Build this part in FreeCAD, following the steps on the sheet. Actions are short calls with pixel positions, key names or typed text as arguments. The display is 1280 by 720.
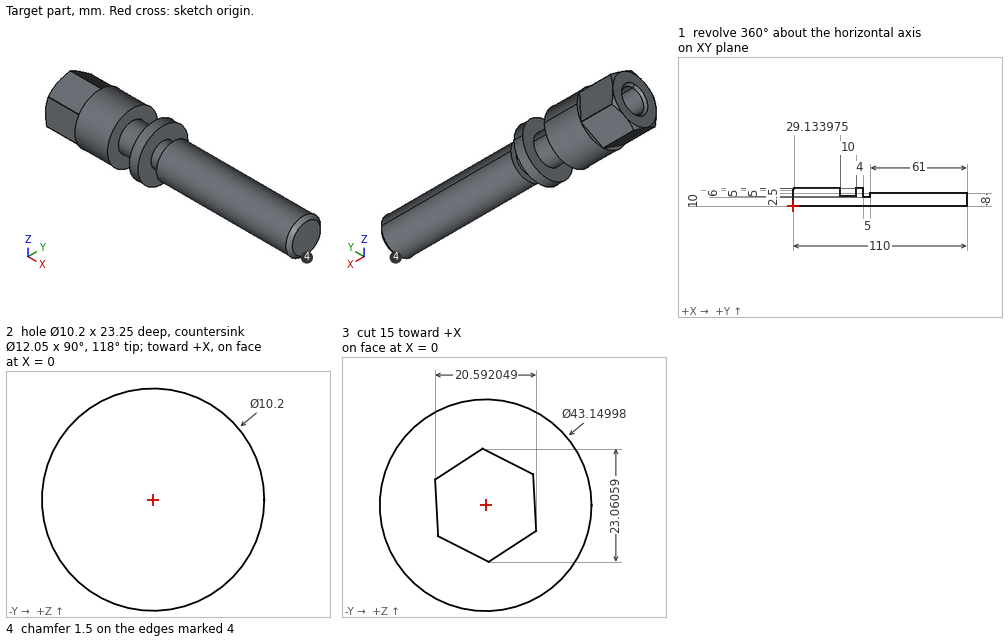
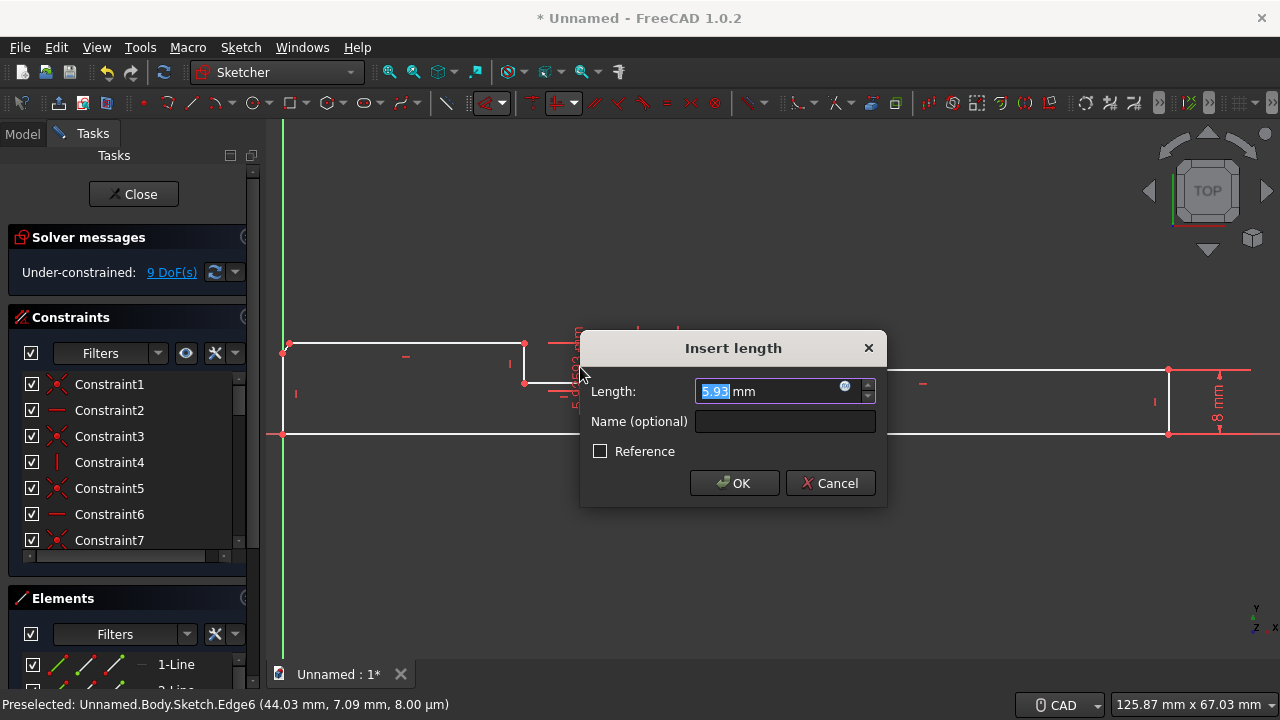
text(6)
key(Return)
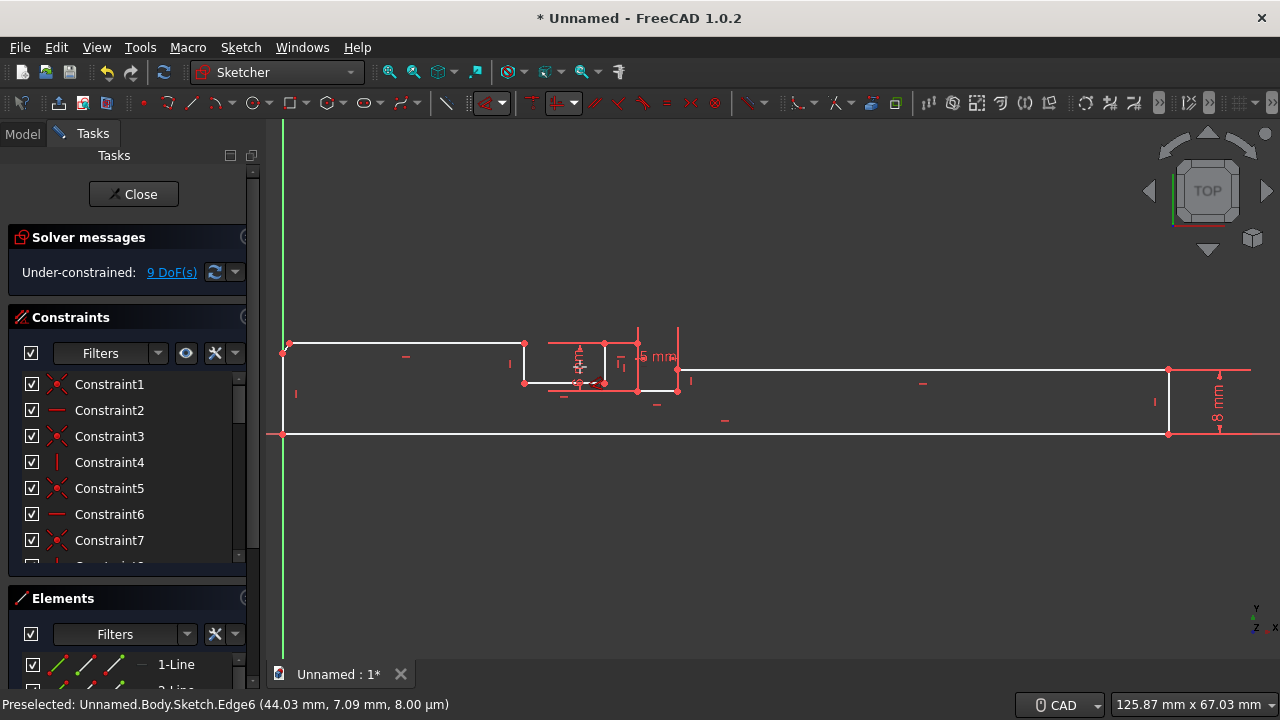
scroll(628, 343, up, 2)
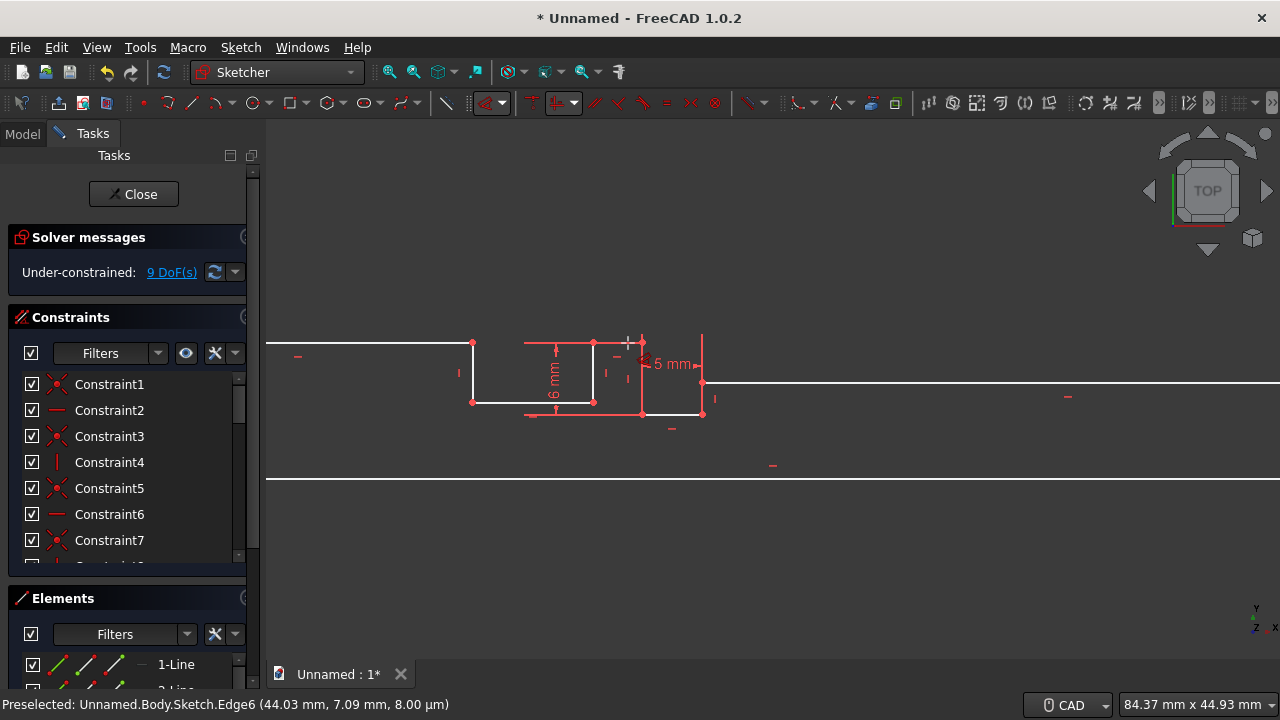
click(627, 343)
click(618, 309)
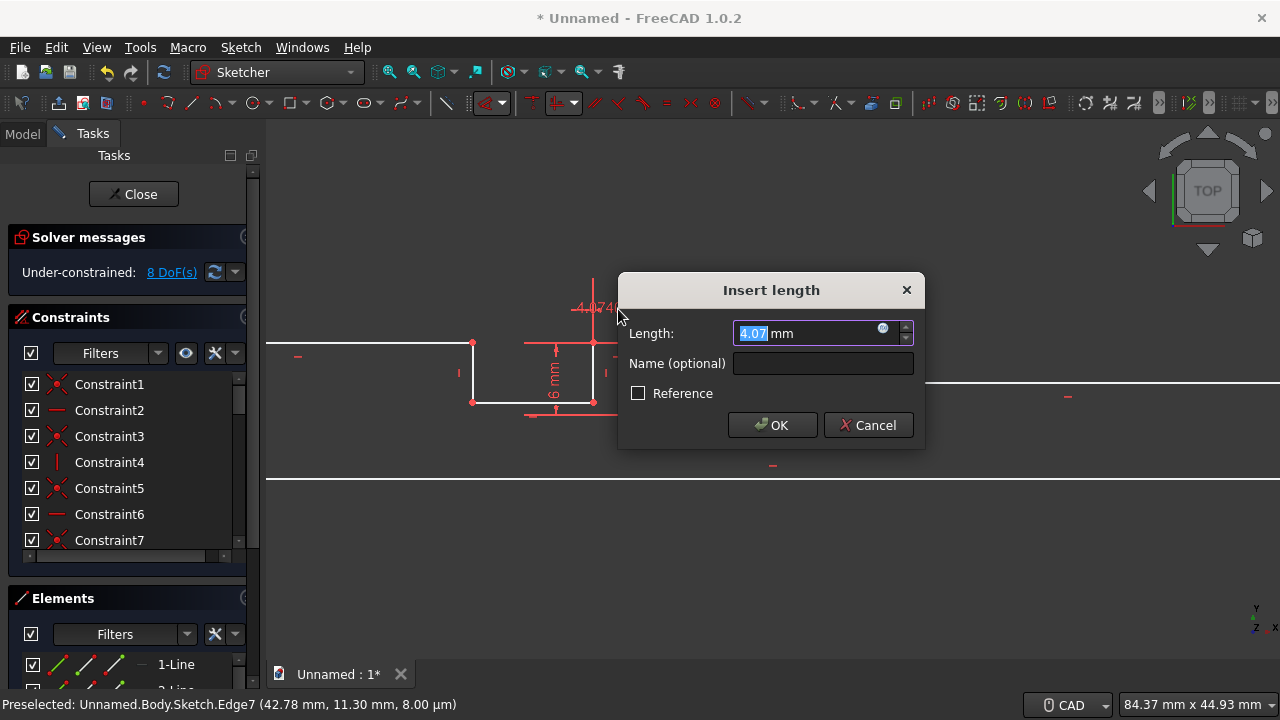
text(4)
key(Return)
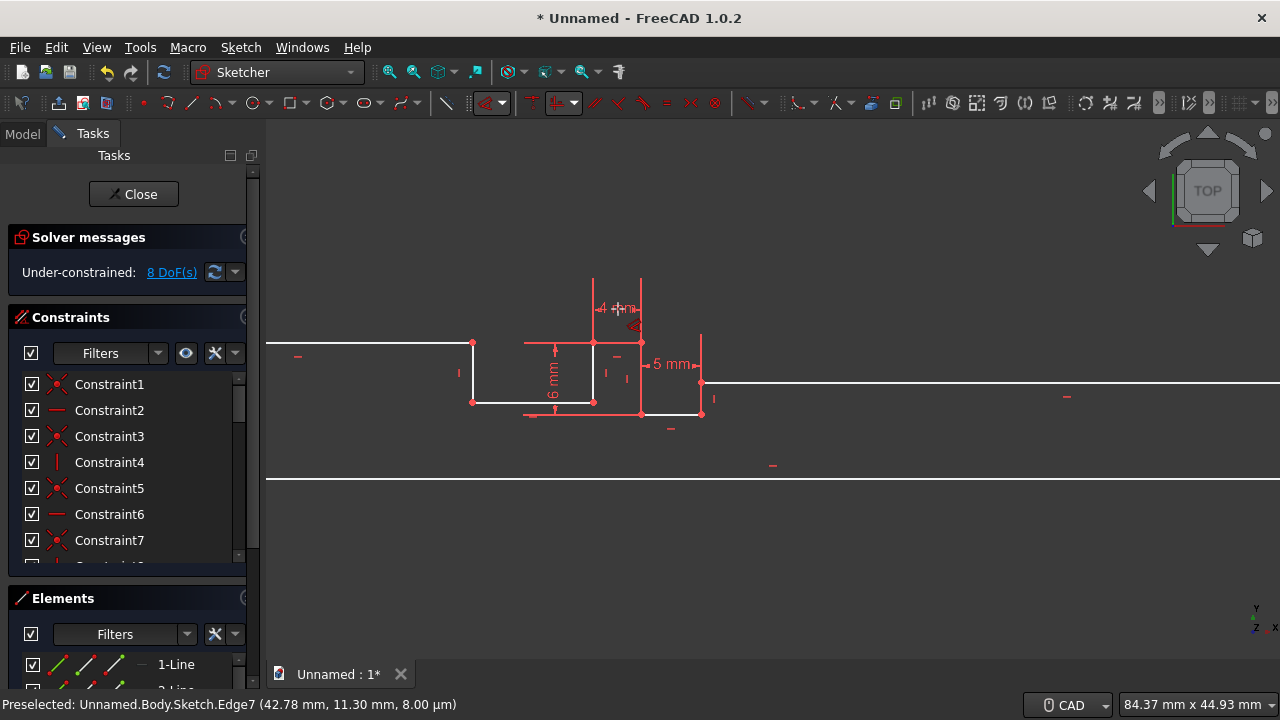
click(593, 361)
click(559, 352)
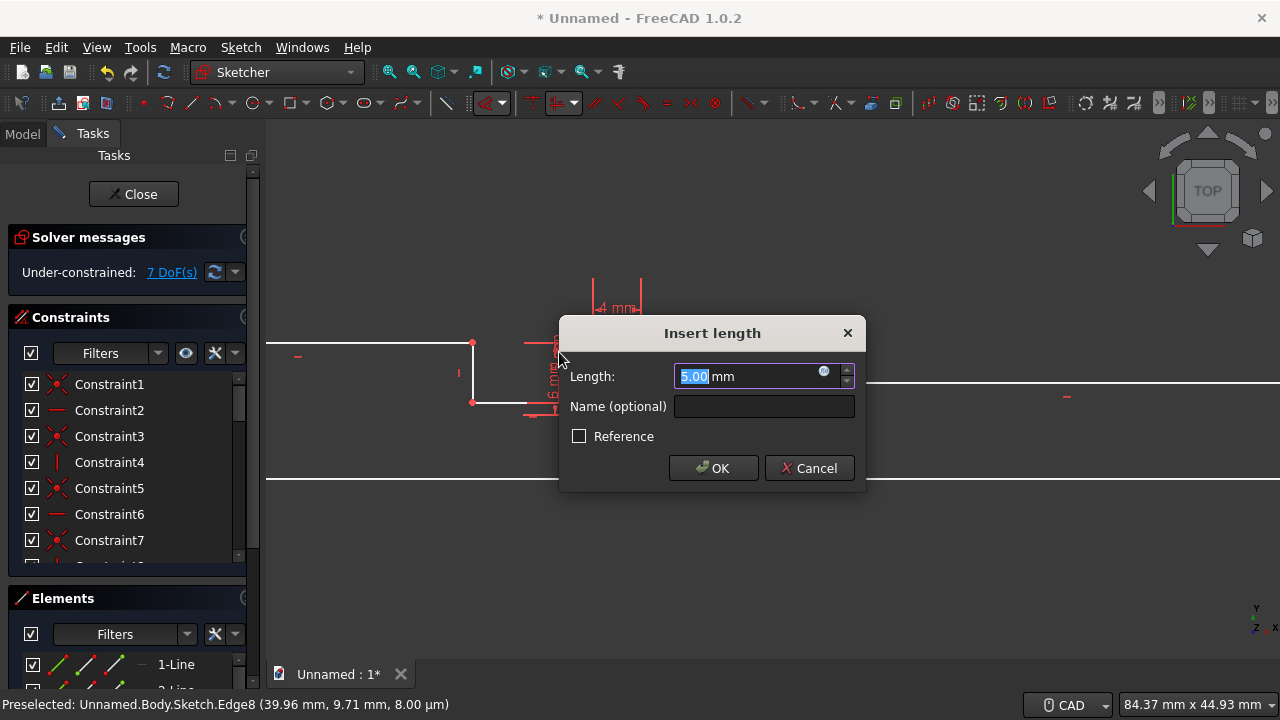
text(5)
key(Return)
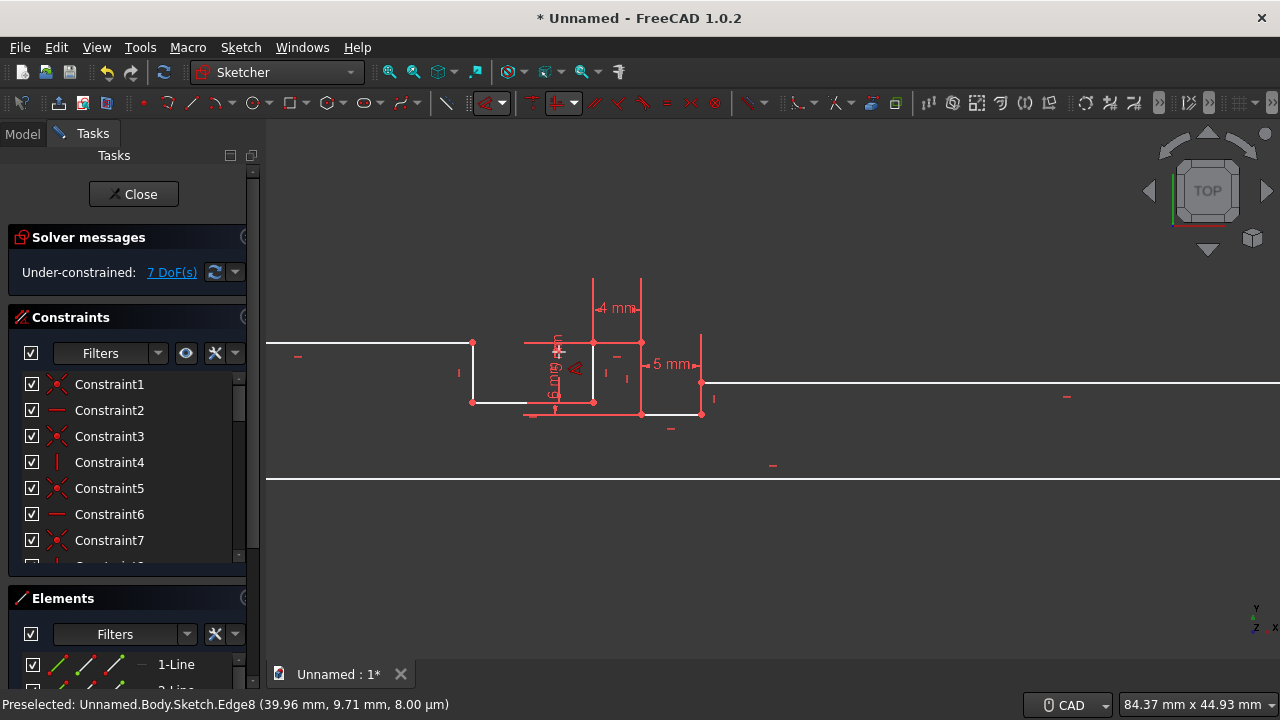
click(473, 385)
click(439, 373)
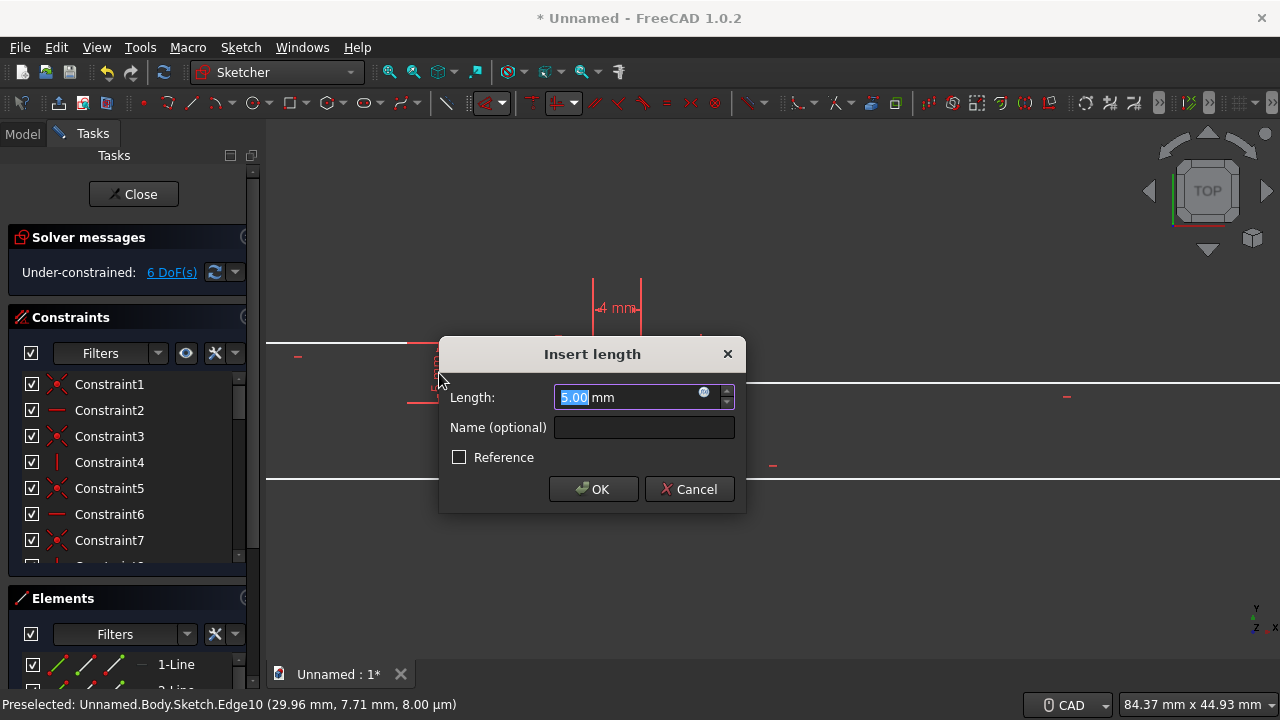
text(5)
key(Return)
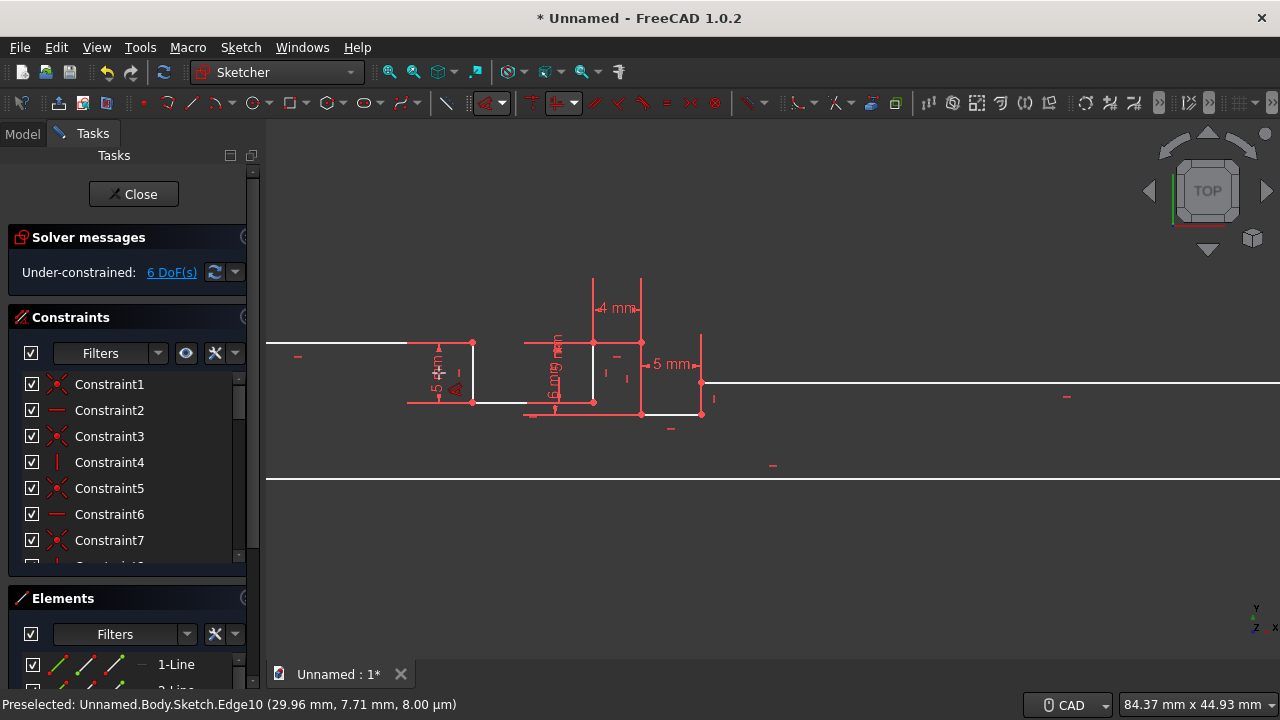
click(921, 383)
click(908, 349)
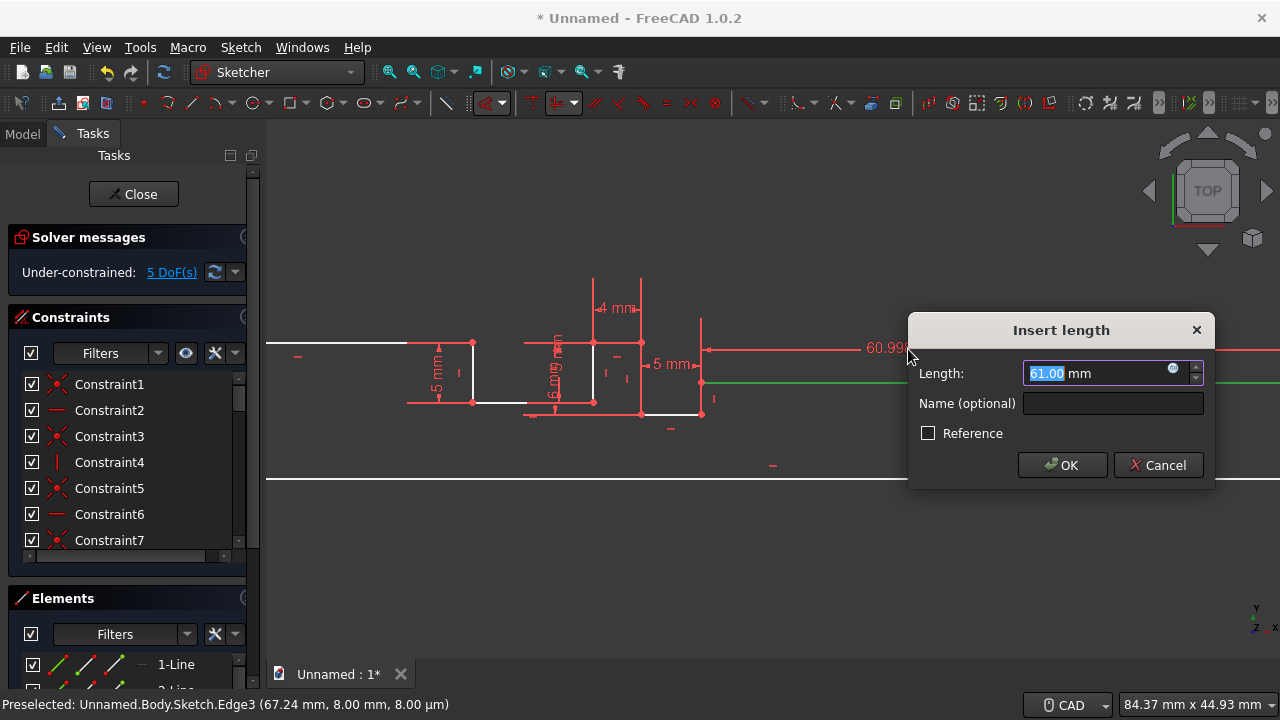
text(61)
key(Return)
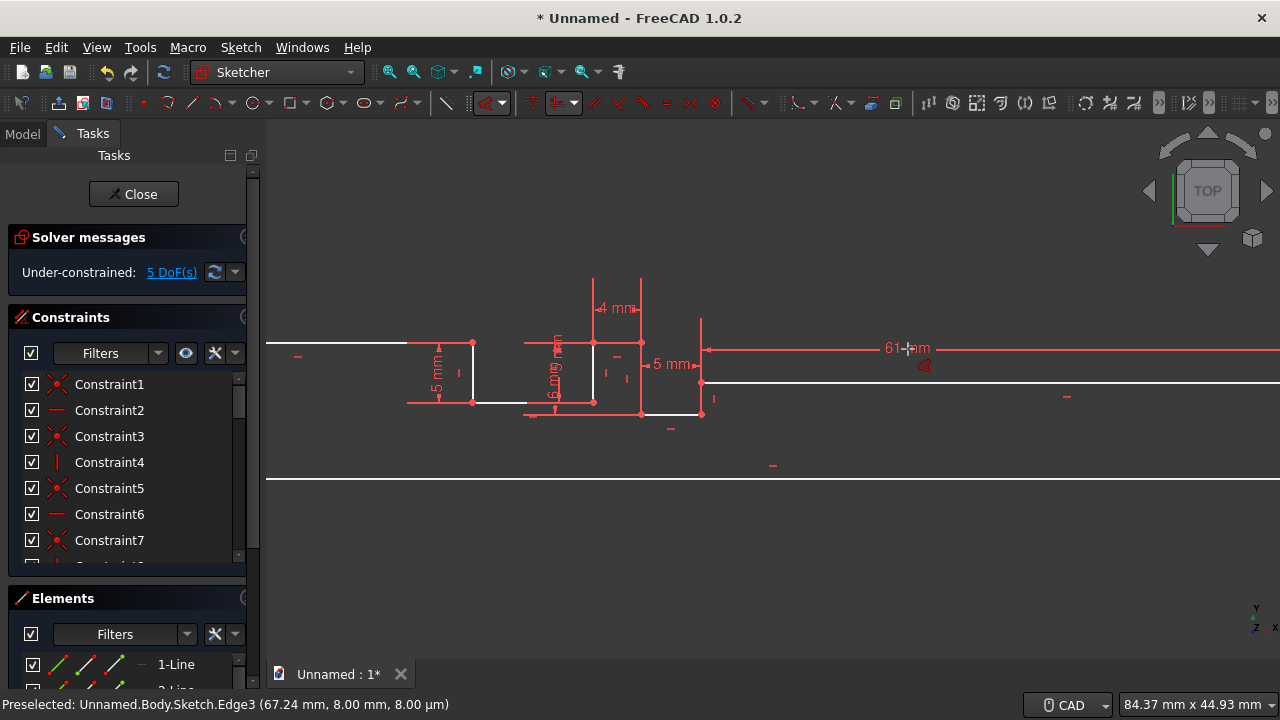
click(557, 403)
click(533, 437)